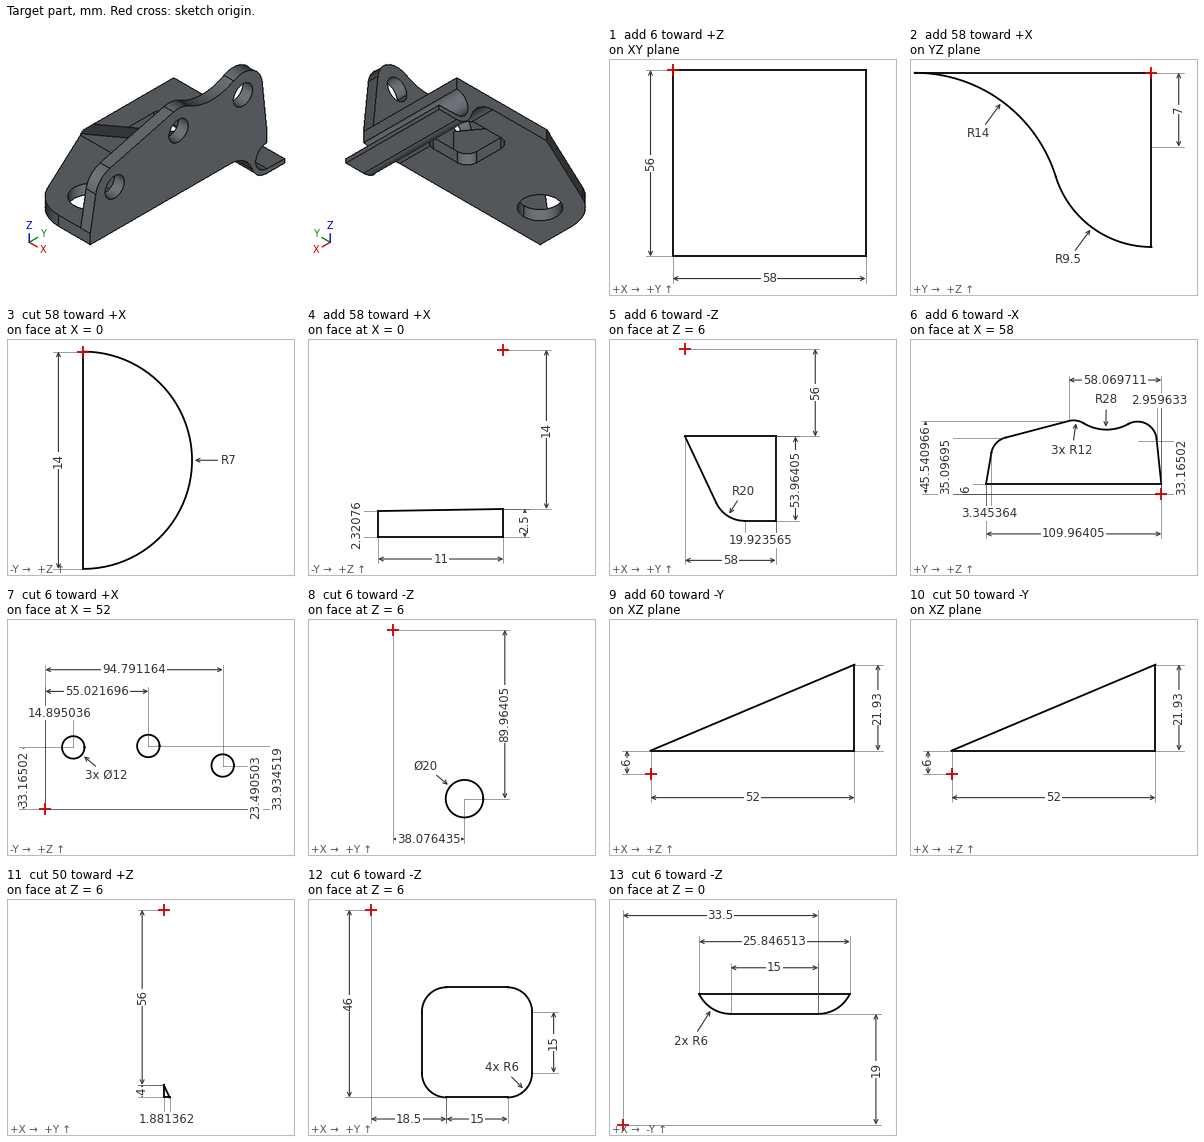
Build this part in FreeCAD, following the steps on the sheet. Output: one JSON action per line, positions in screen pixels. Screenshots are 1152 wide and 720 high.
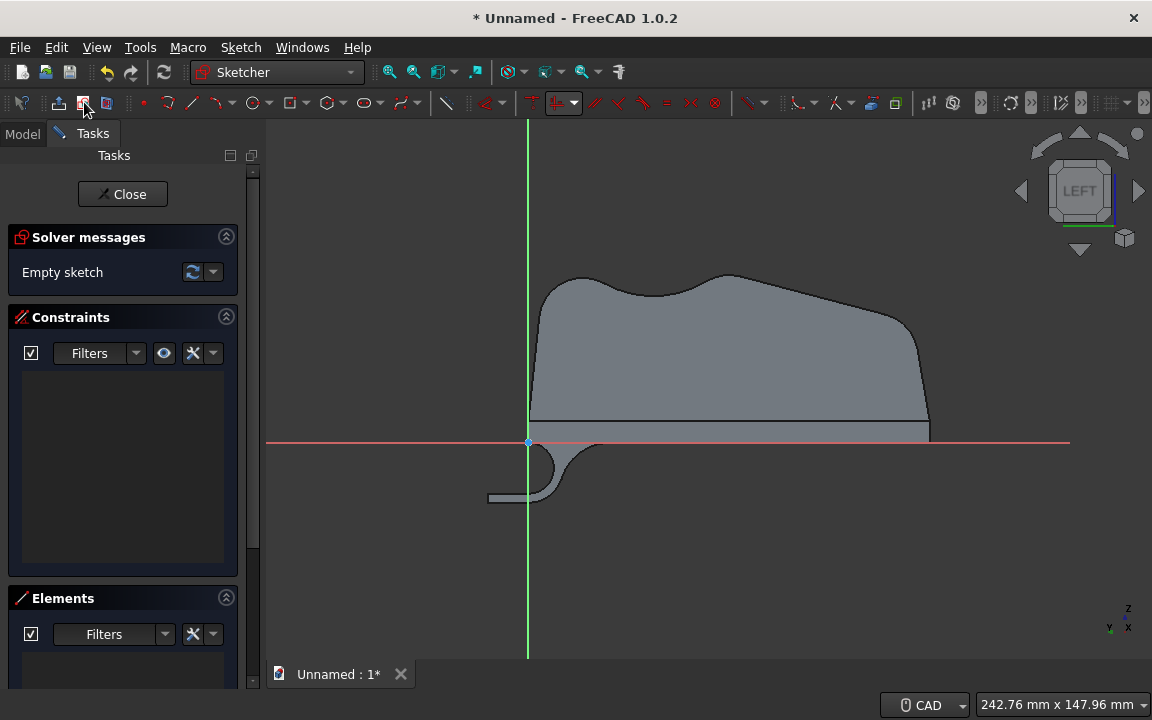
{"action": "left_click", "coordinate": [254, 104]}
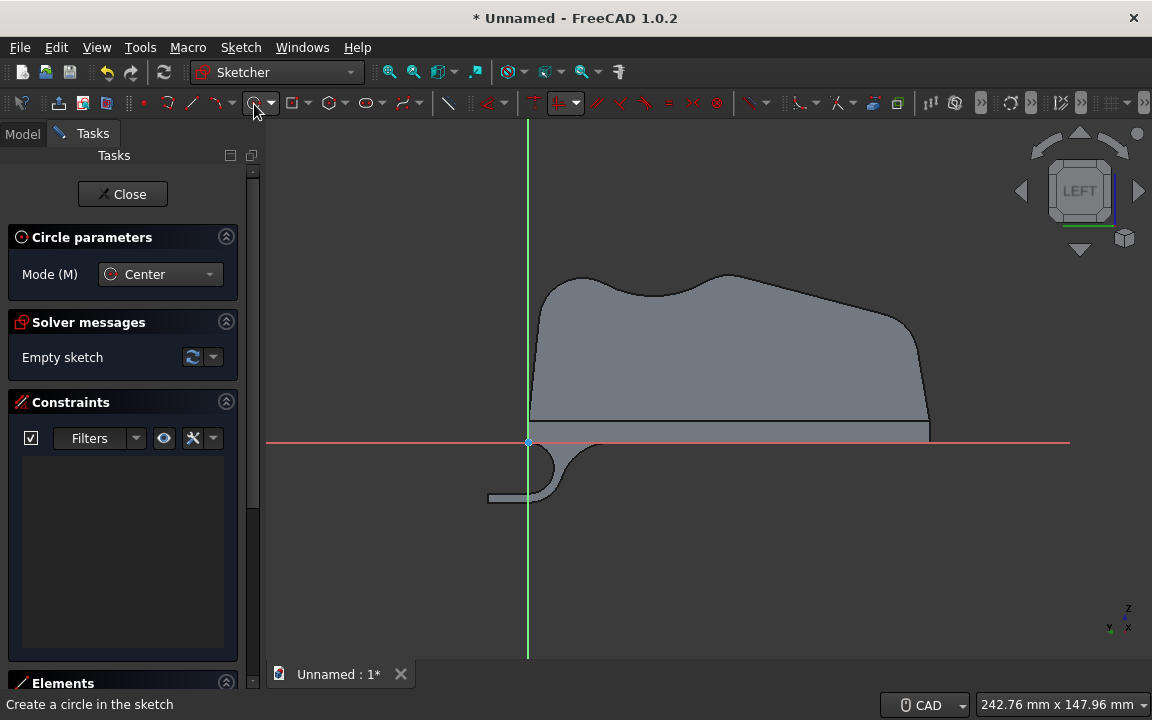
{"action": "left_click", "coordinate": [583, 322]}
{"action": "left_click", "coordinate": [598, 306]}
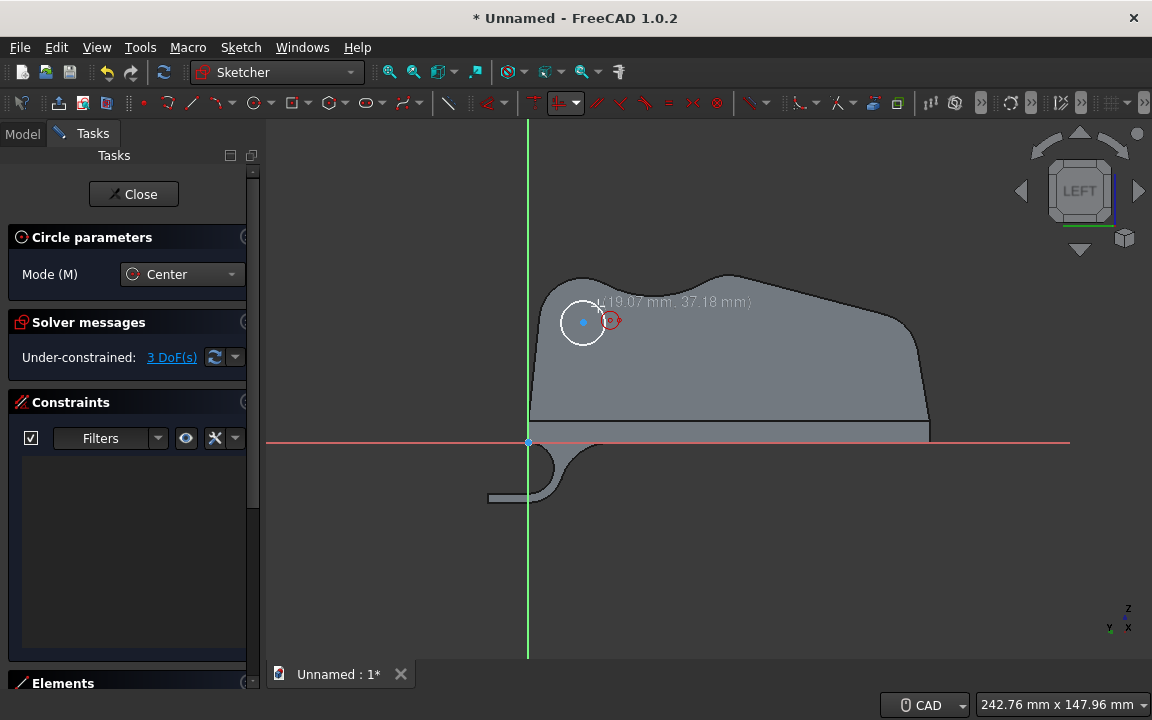
{"action": "left_click", "coordinate": [729, 319]}
{"action": "left_click", "coordinate": [745, 303]}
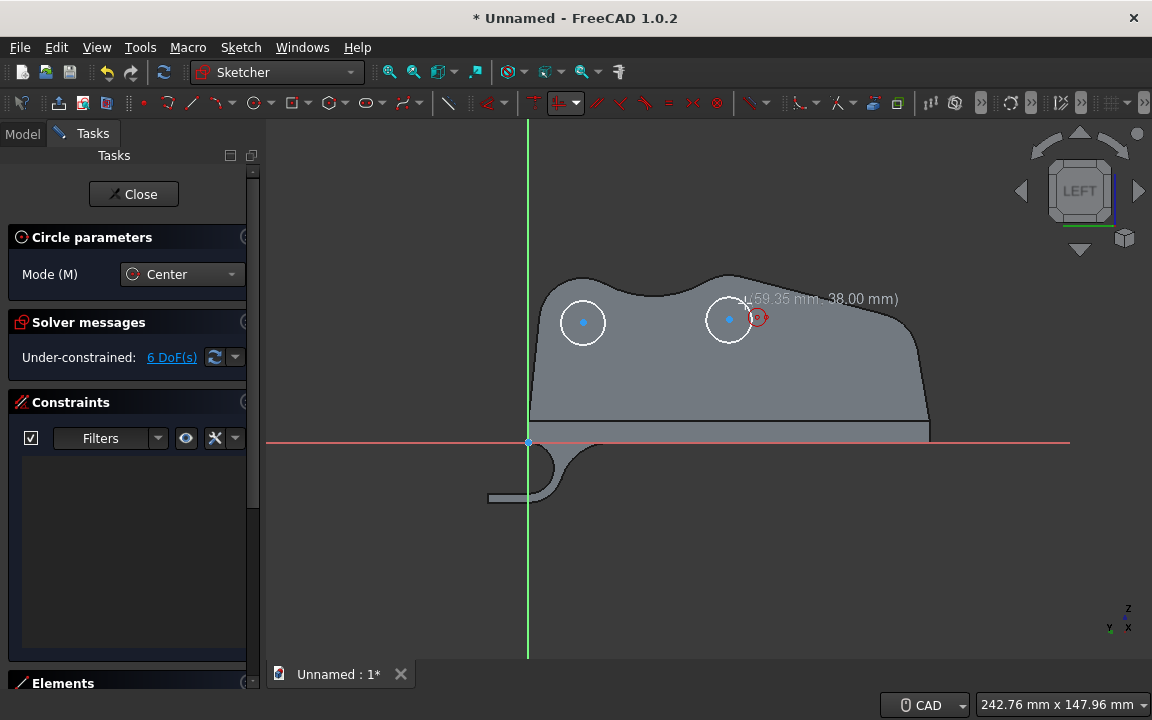
{"action": "left_click", "coordinate": [874, 357]}
{"action": "left_click", "coordinate": [890, 341]}
{"action": "key", "text": "Escape"}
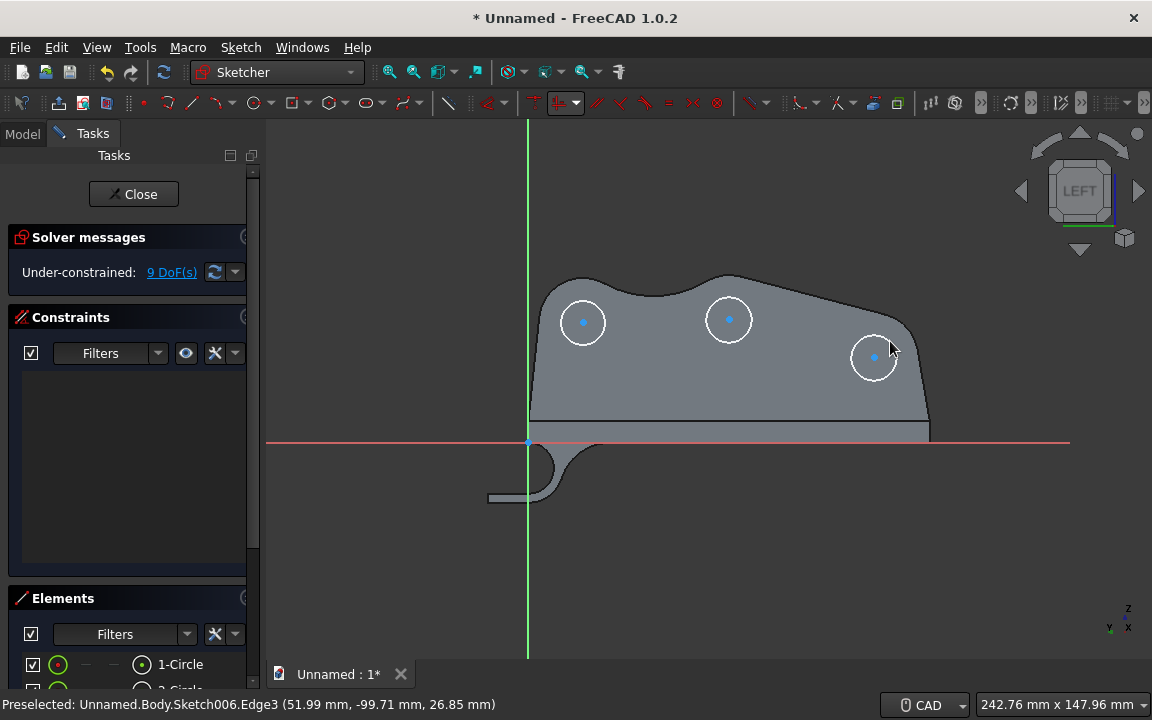
{"action": "left_click", "coordinate": [598, 307]}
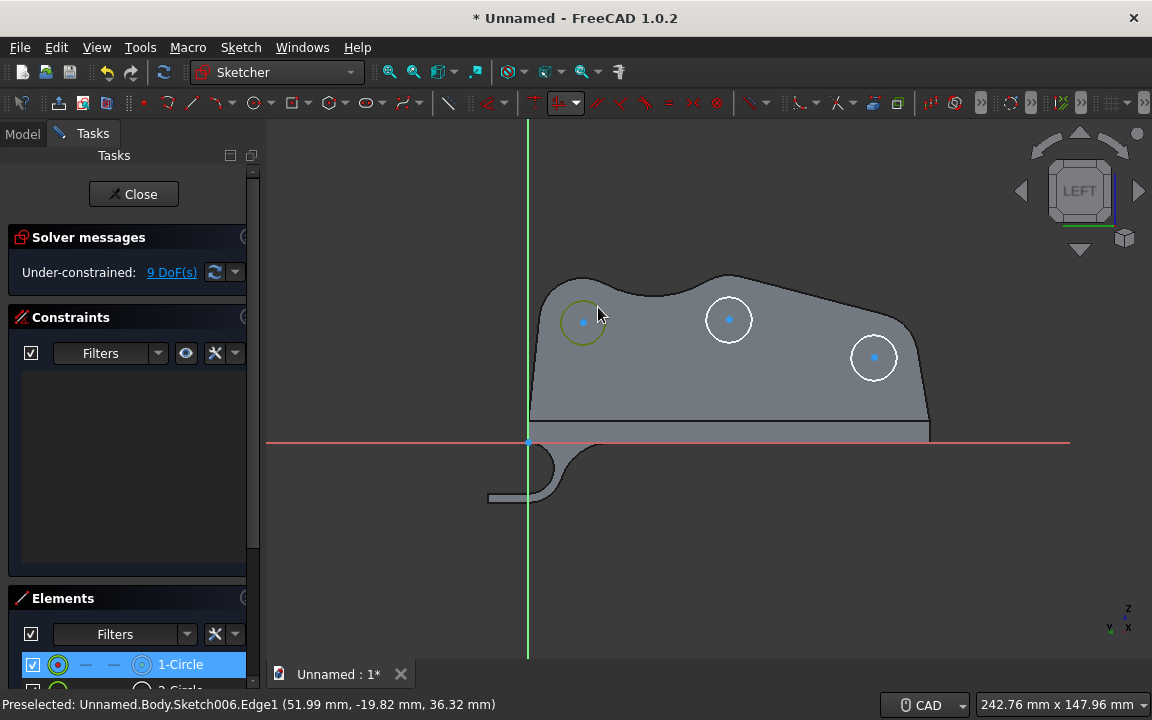
{"action": "left_click", "coordinate": [745, 304]}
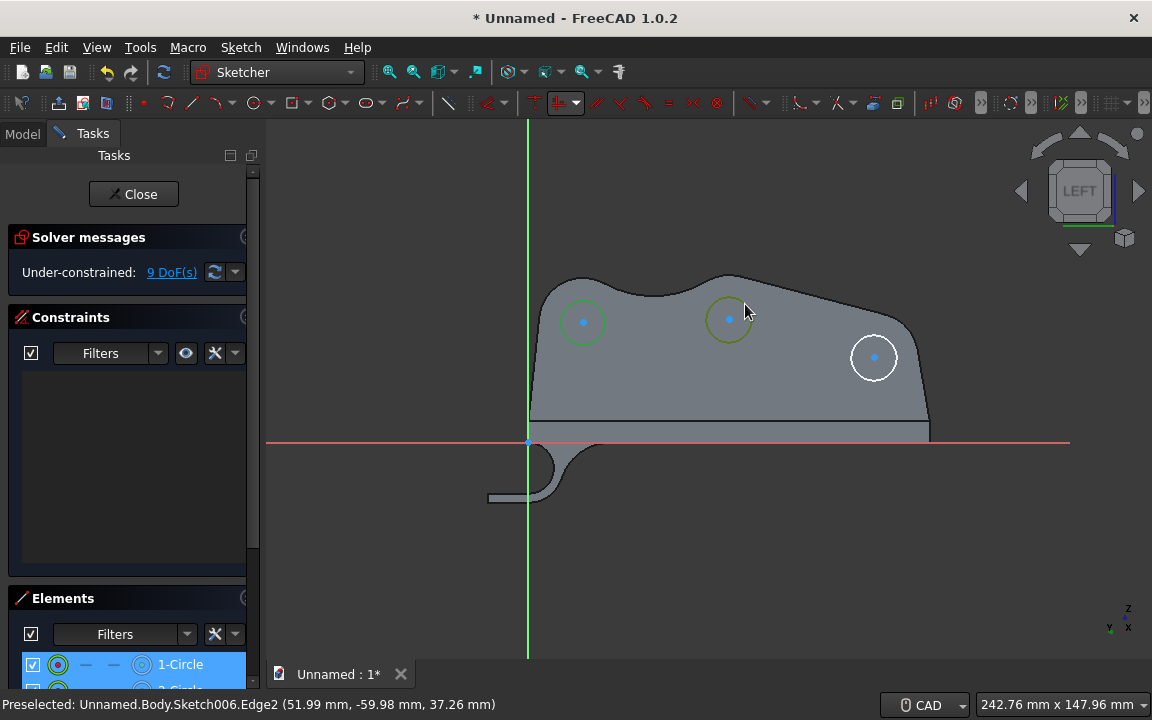
{"action": "left_click", "coordinate": [890, 342]}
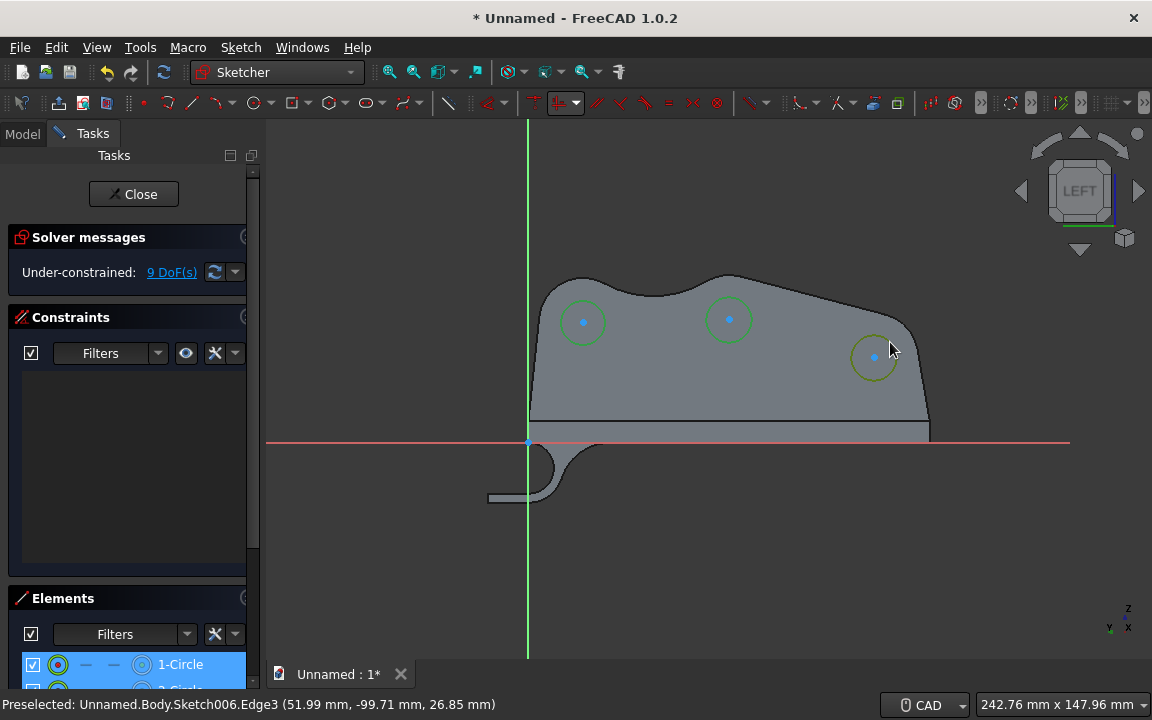
{"action": "left_click", "coordinate": [670, 104]}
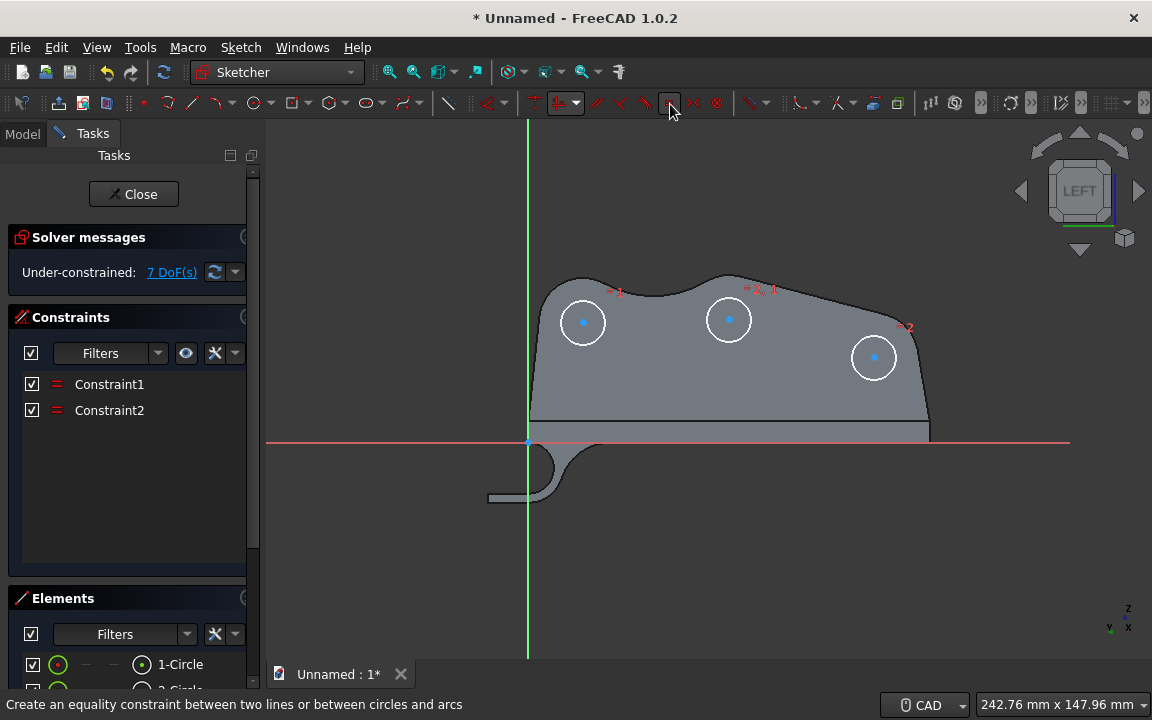
{"action": "key", "text": "d"}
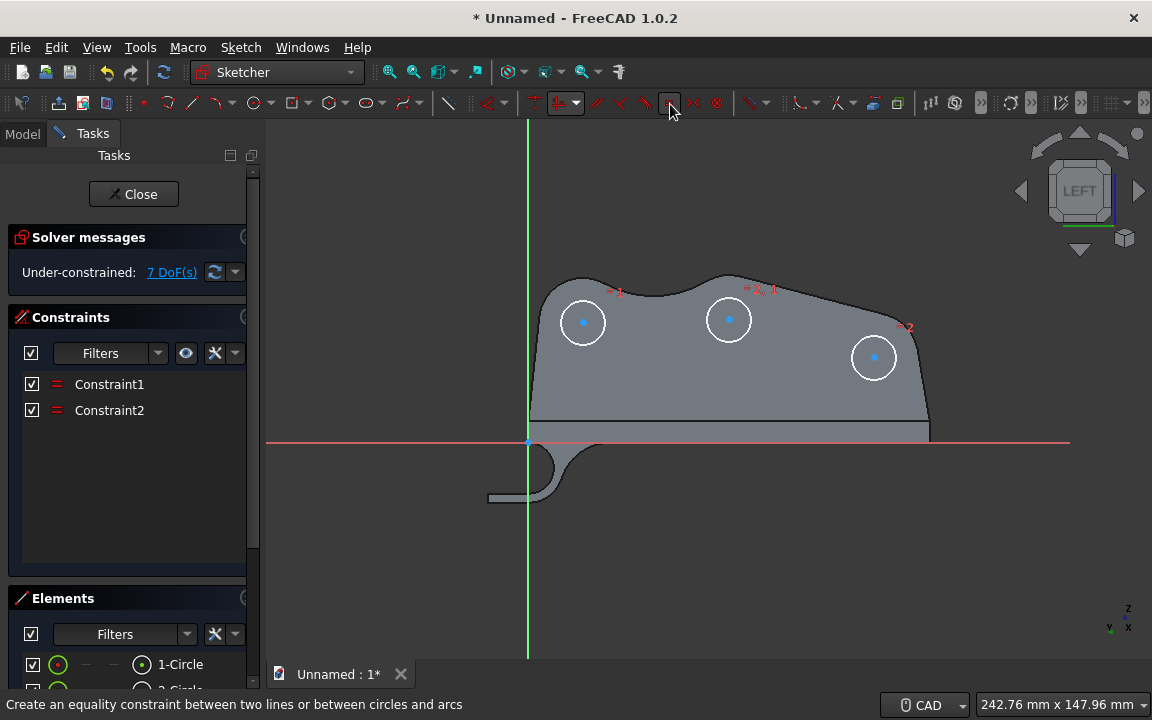
{"action": "left_click", "coordinate": [598, 307]}
{"action": "left_click", "coordinate": [620, 284]}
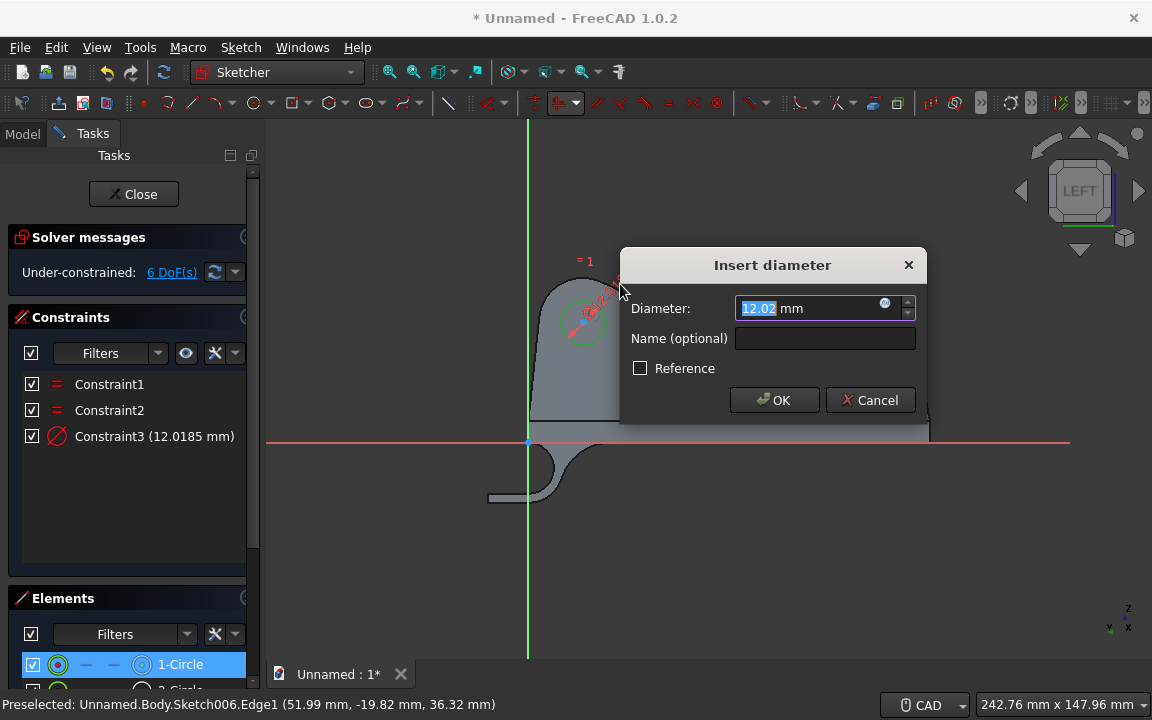
{"action": "type", "text": "12"}
{"action": "key", "text": "Return"}